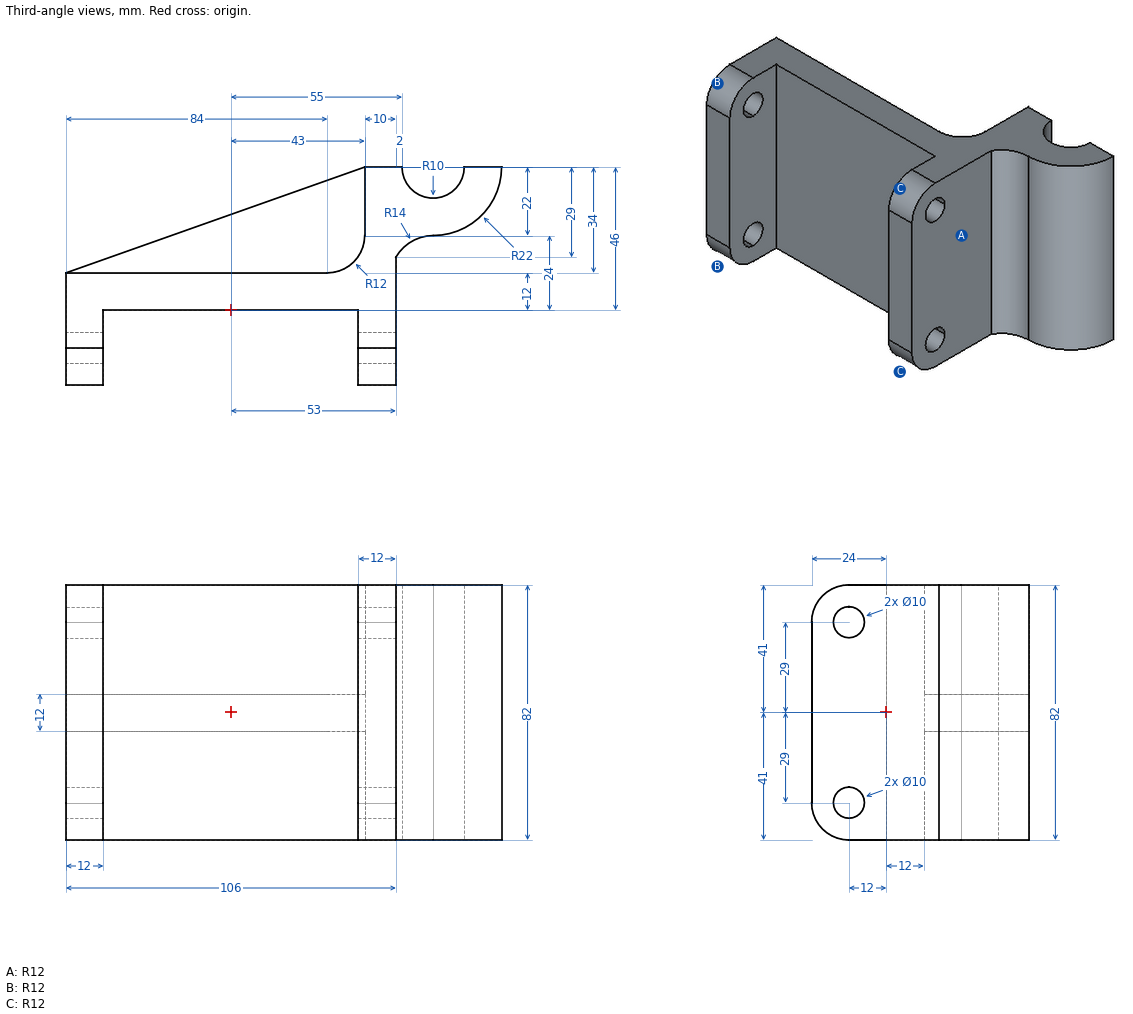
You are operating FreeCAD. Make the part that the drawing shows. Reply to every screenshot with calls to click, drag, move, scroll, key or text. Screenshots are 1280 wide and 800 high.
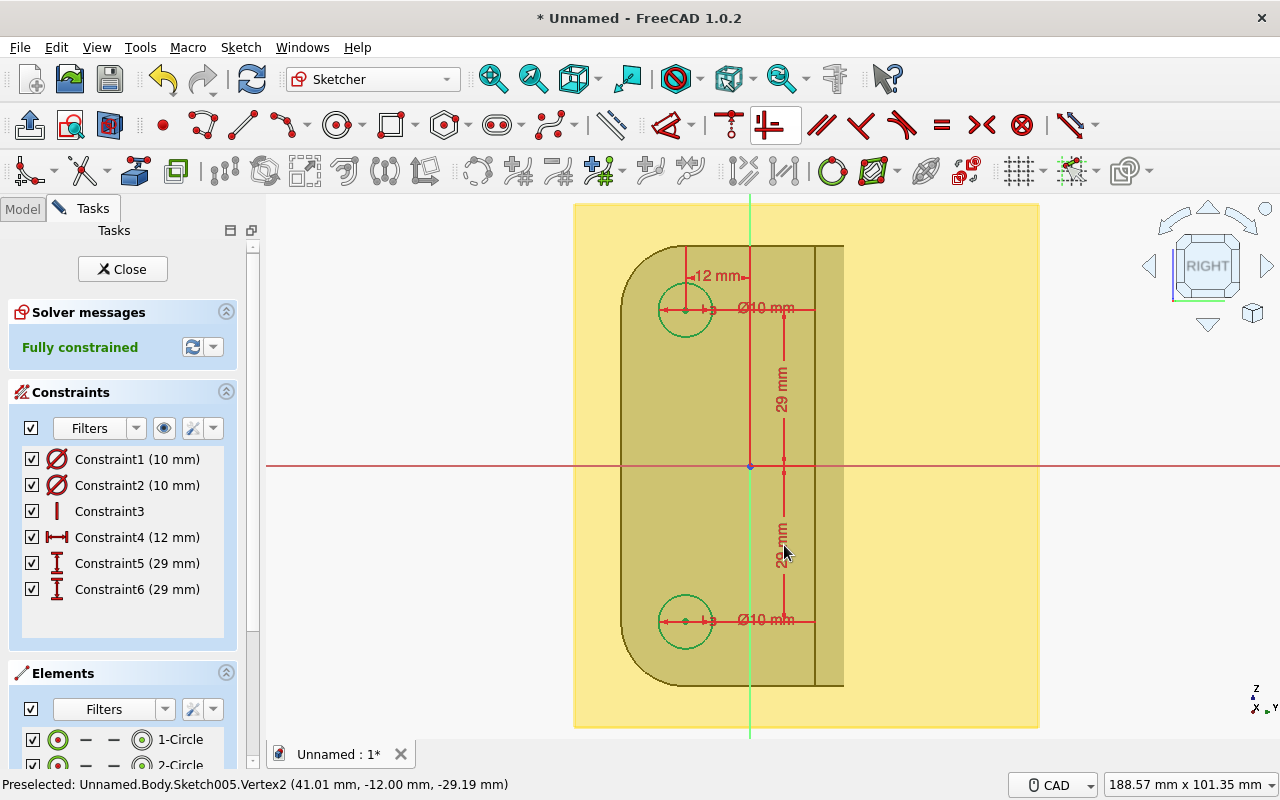
click(123, 269)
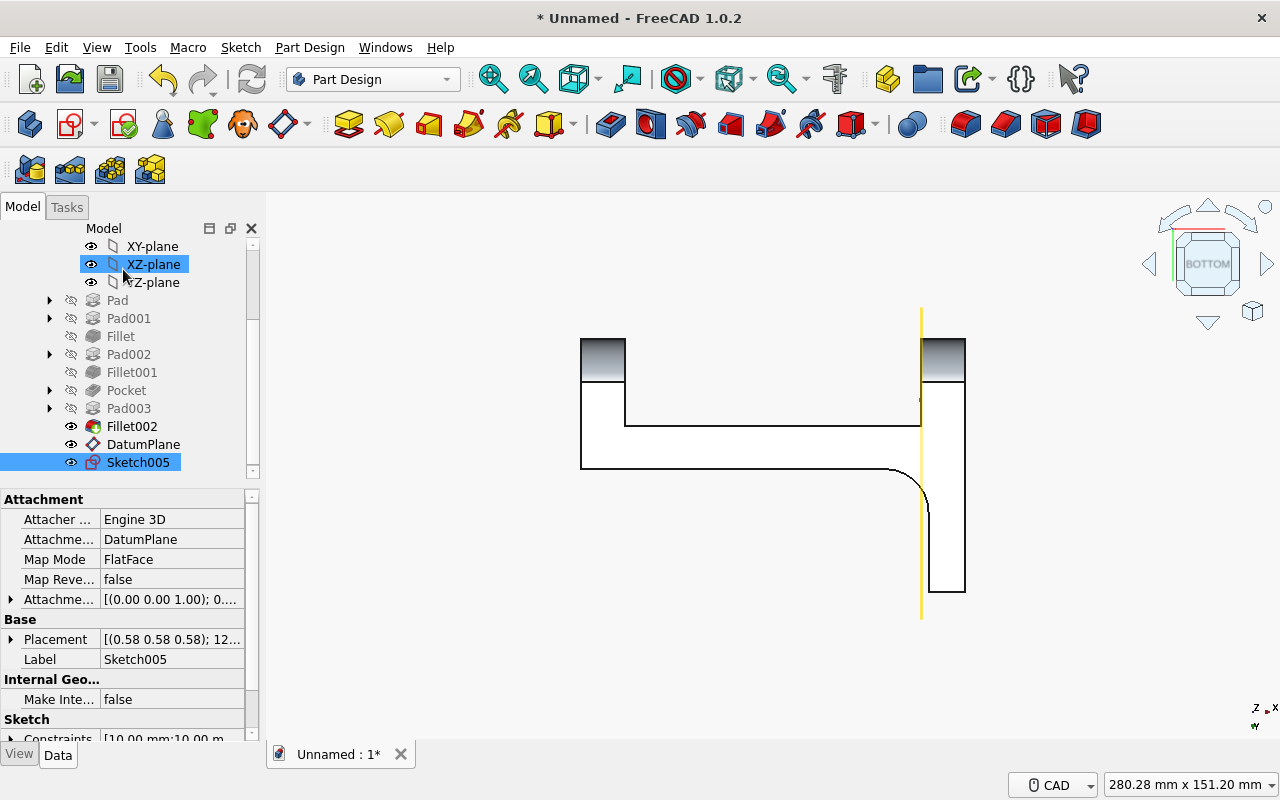
click(612, 124)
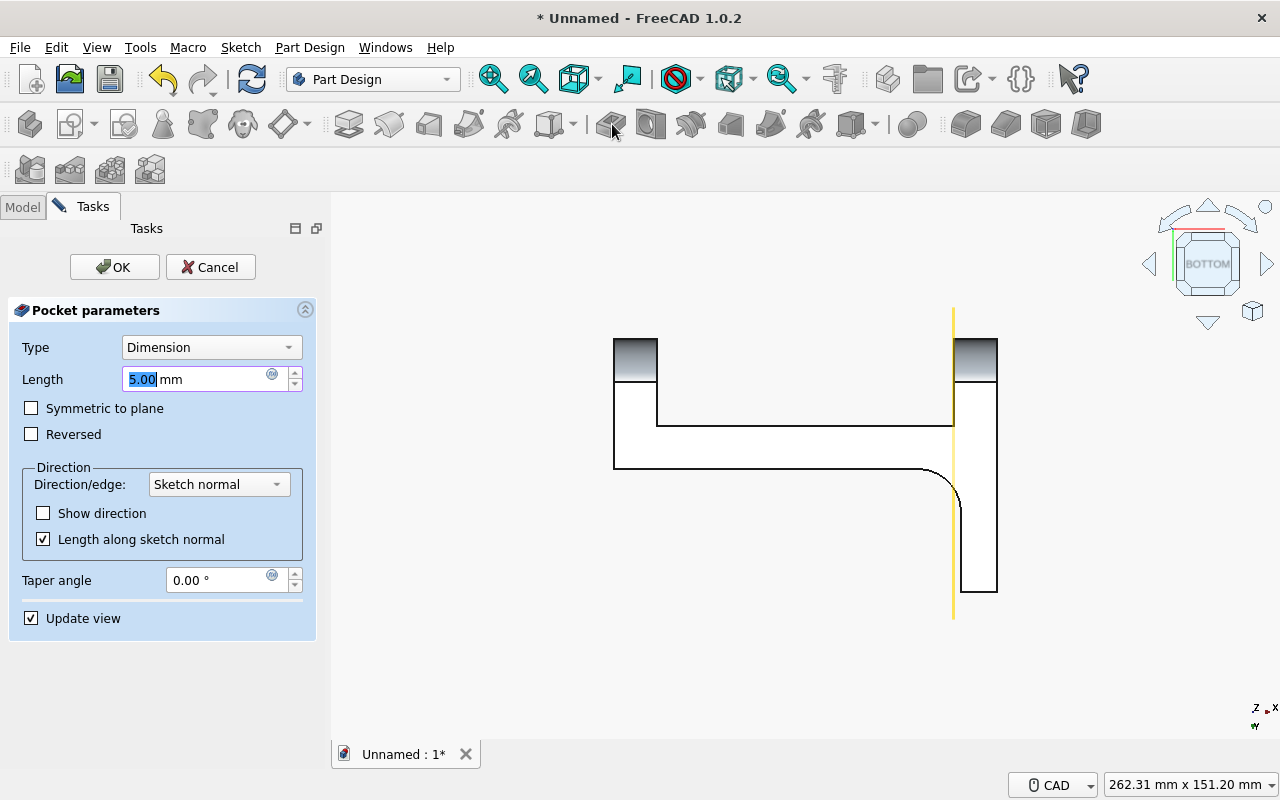
text(12)
key(Tab)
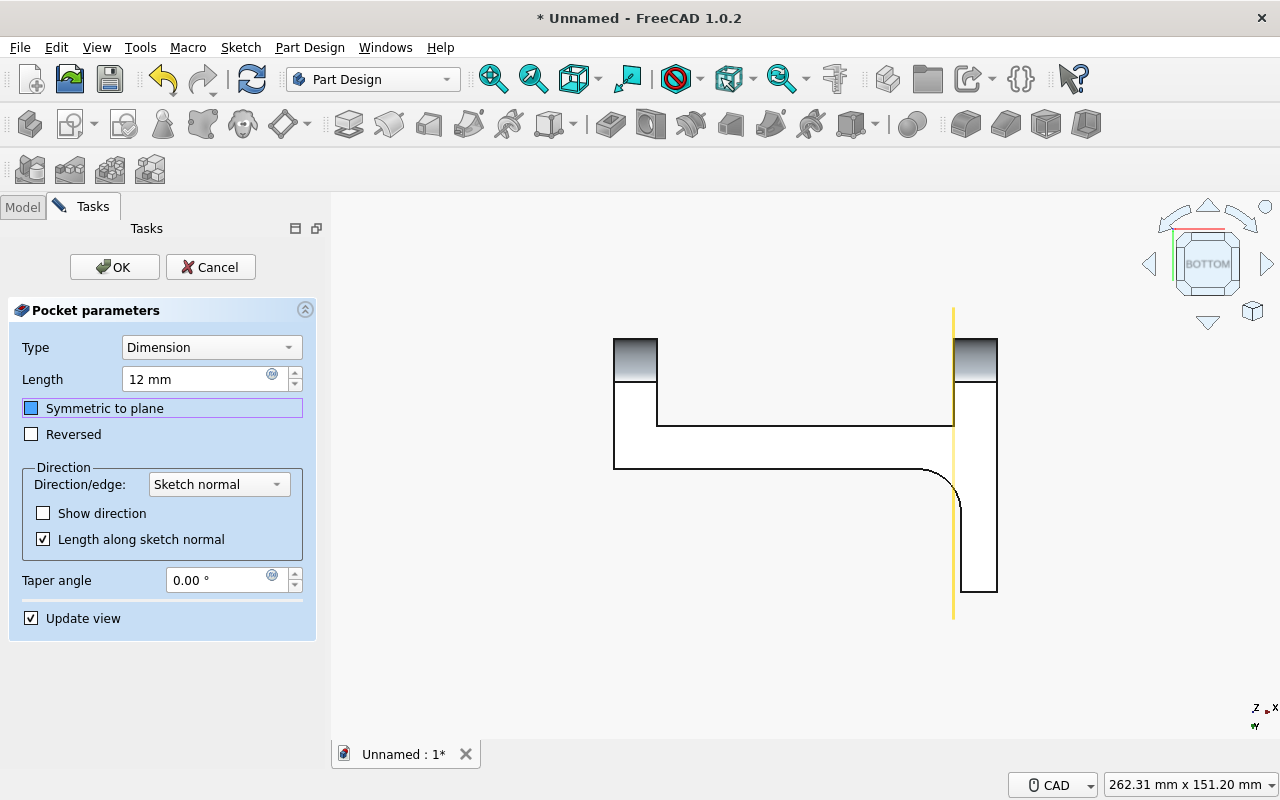
click(30, 434)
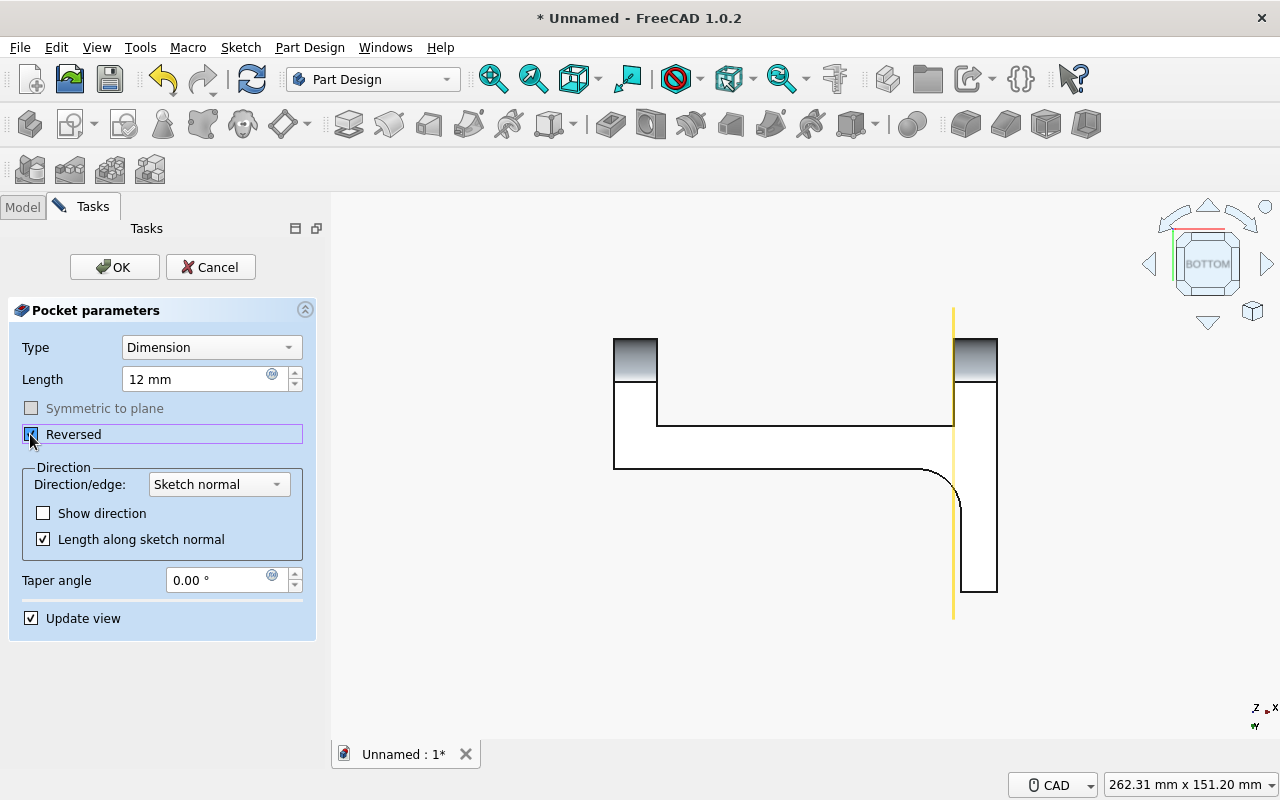
click(115, 267)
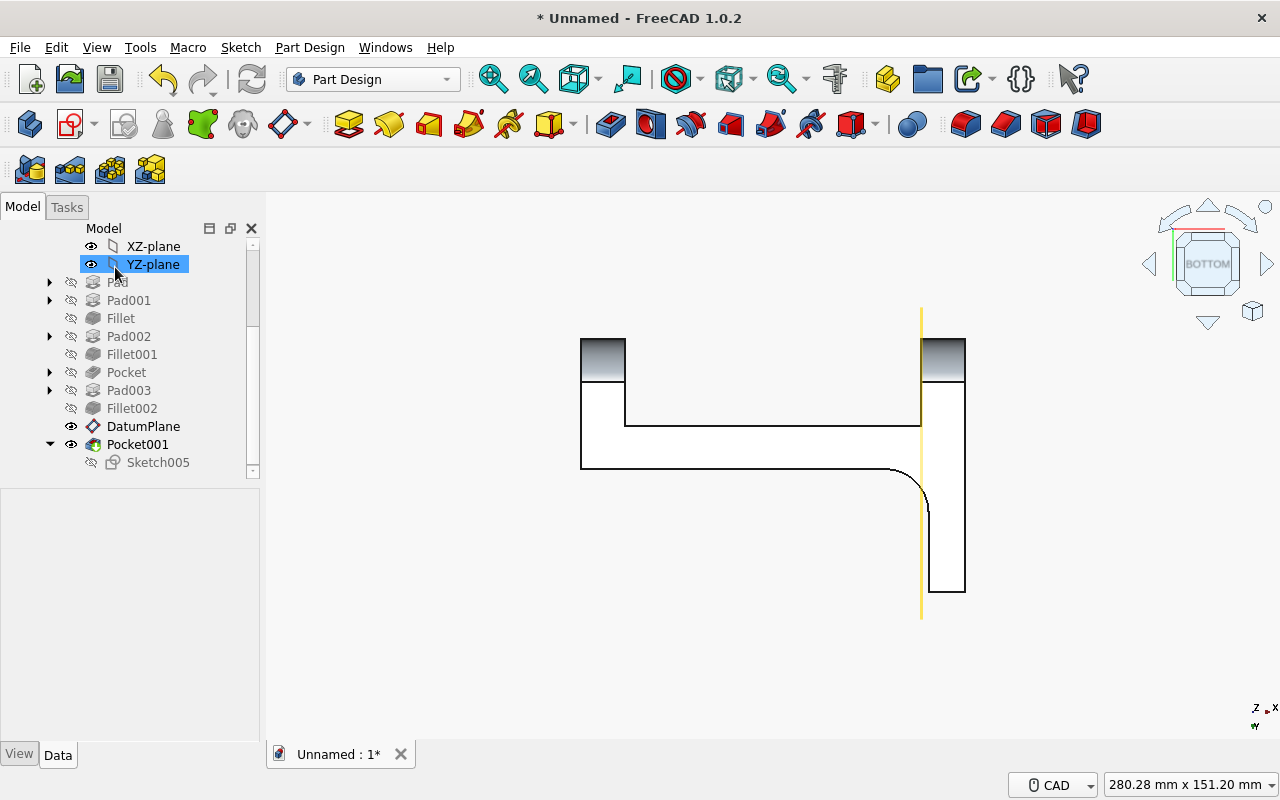
click(116, 426)
key(space)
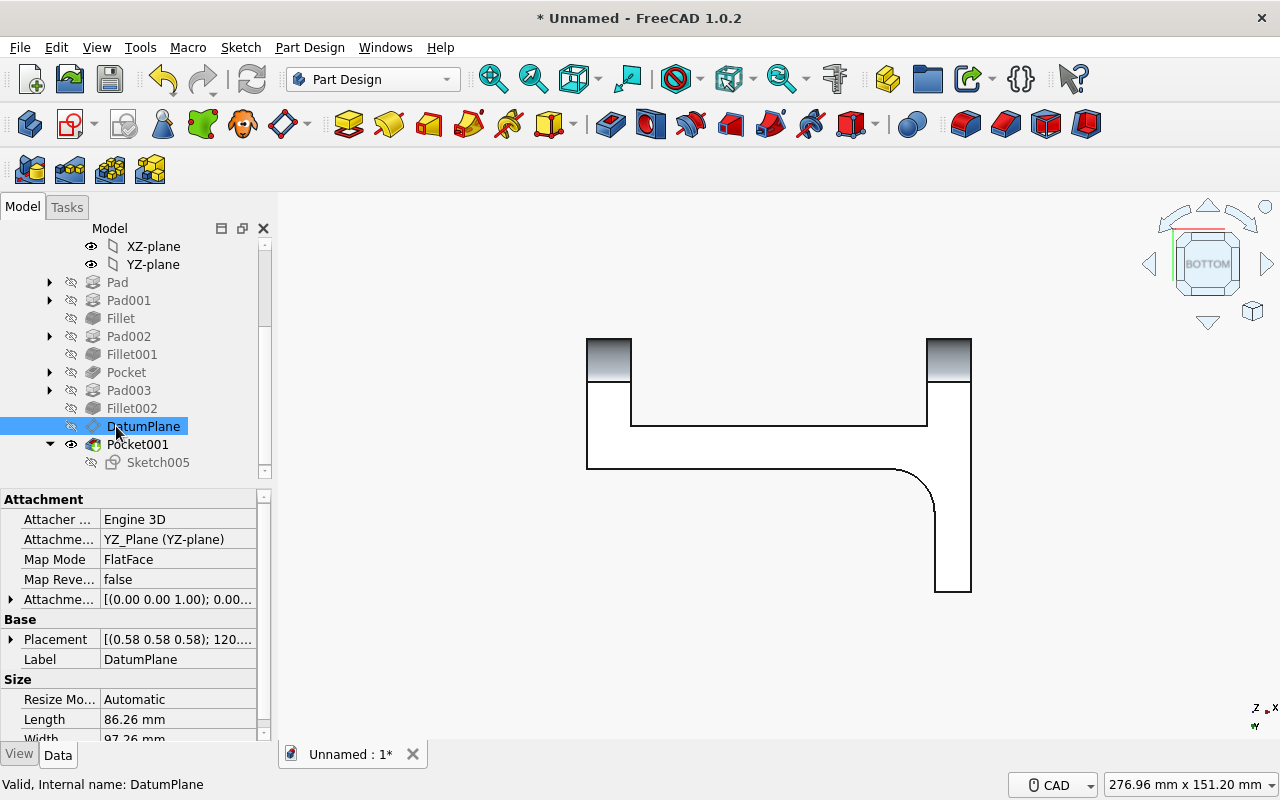
click(318, 699)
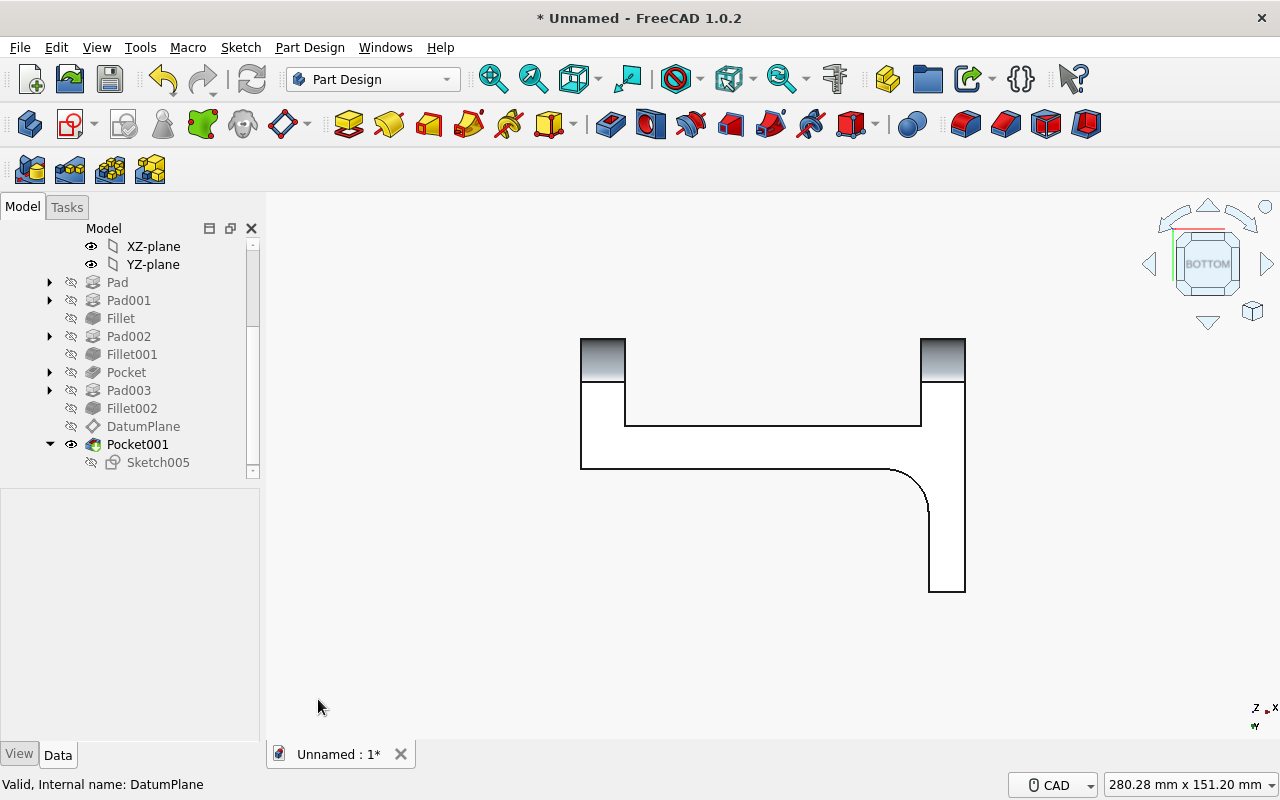
click(70, 124)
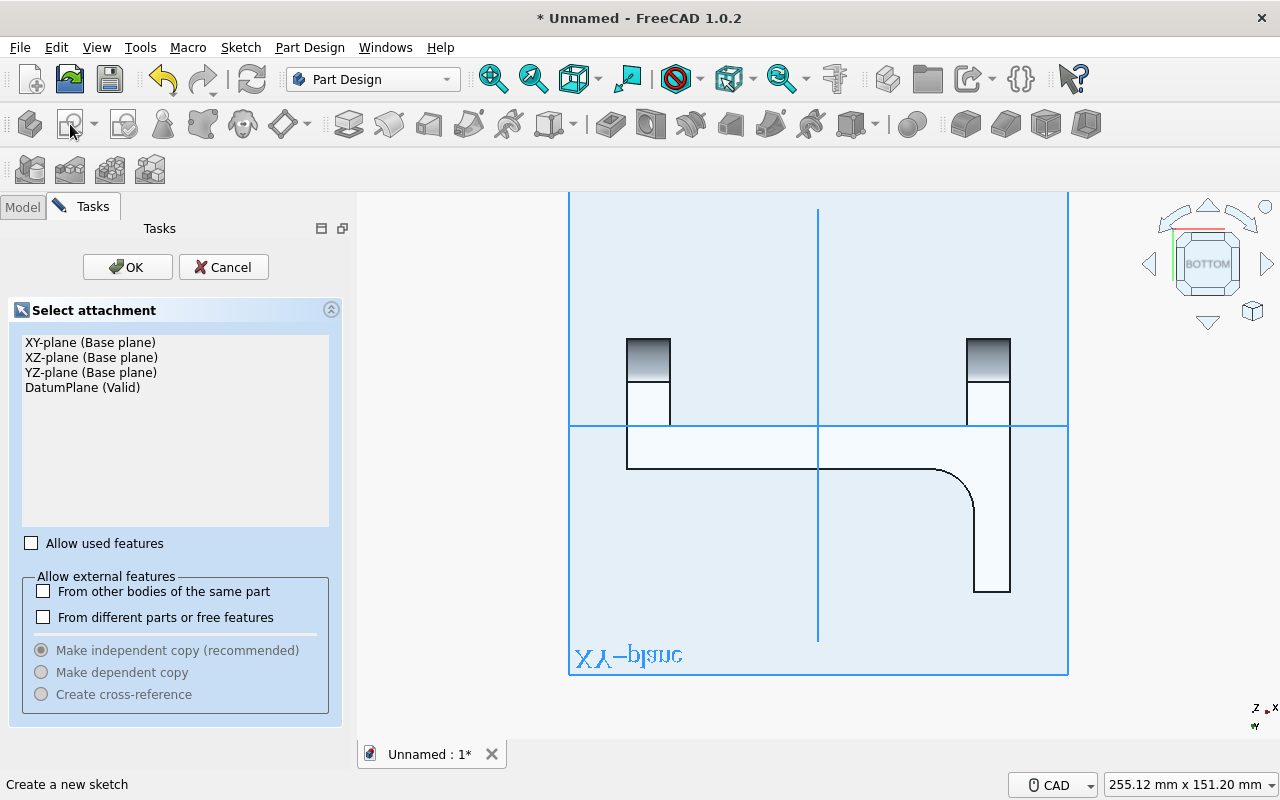
click(82, 342)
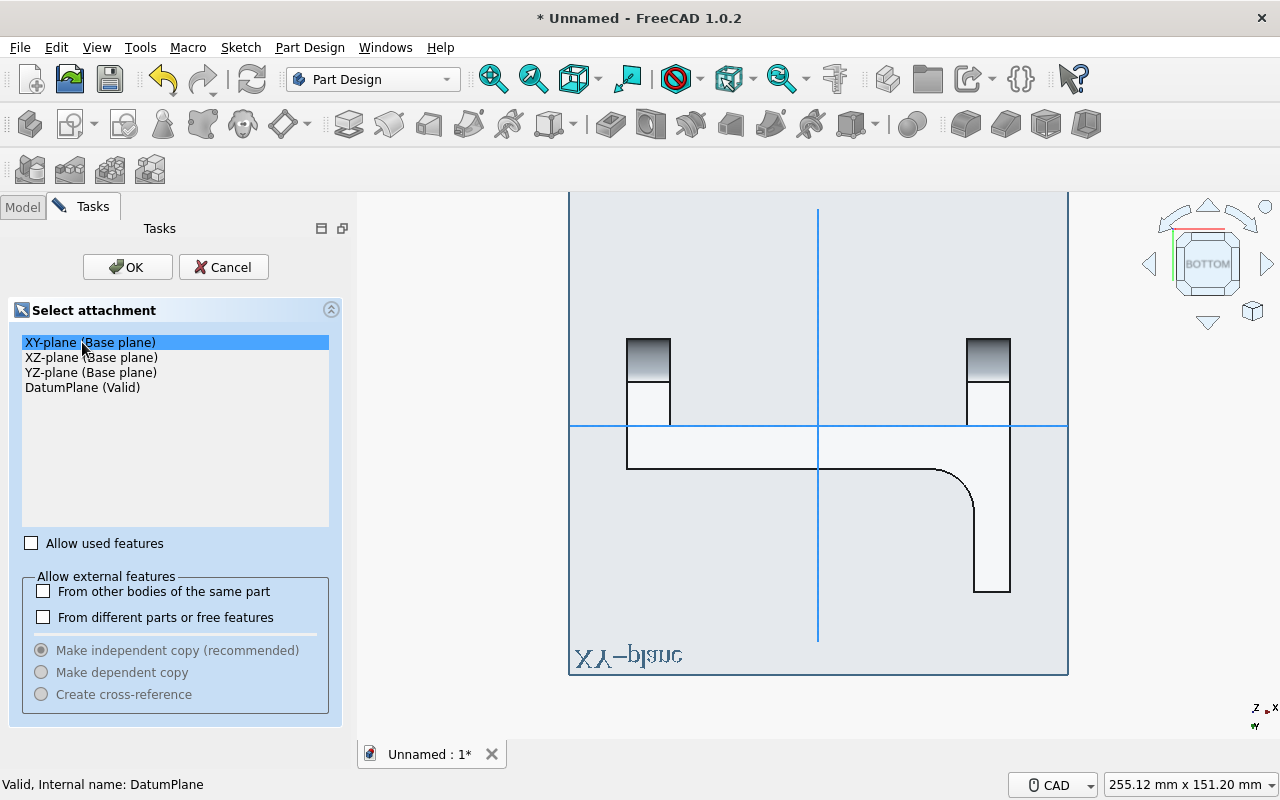
click(128, 267)